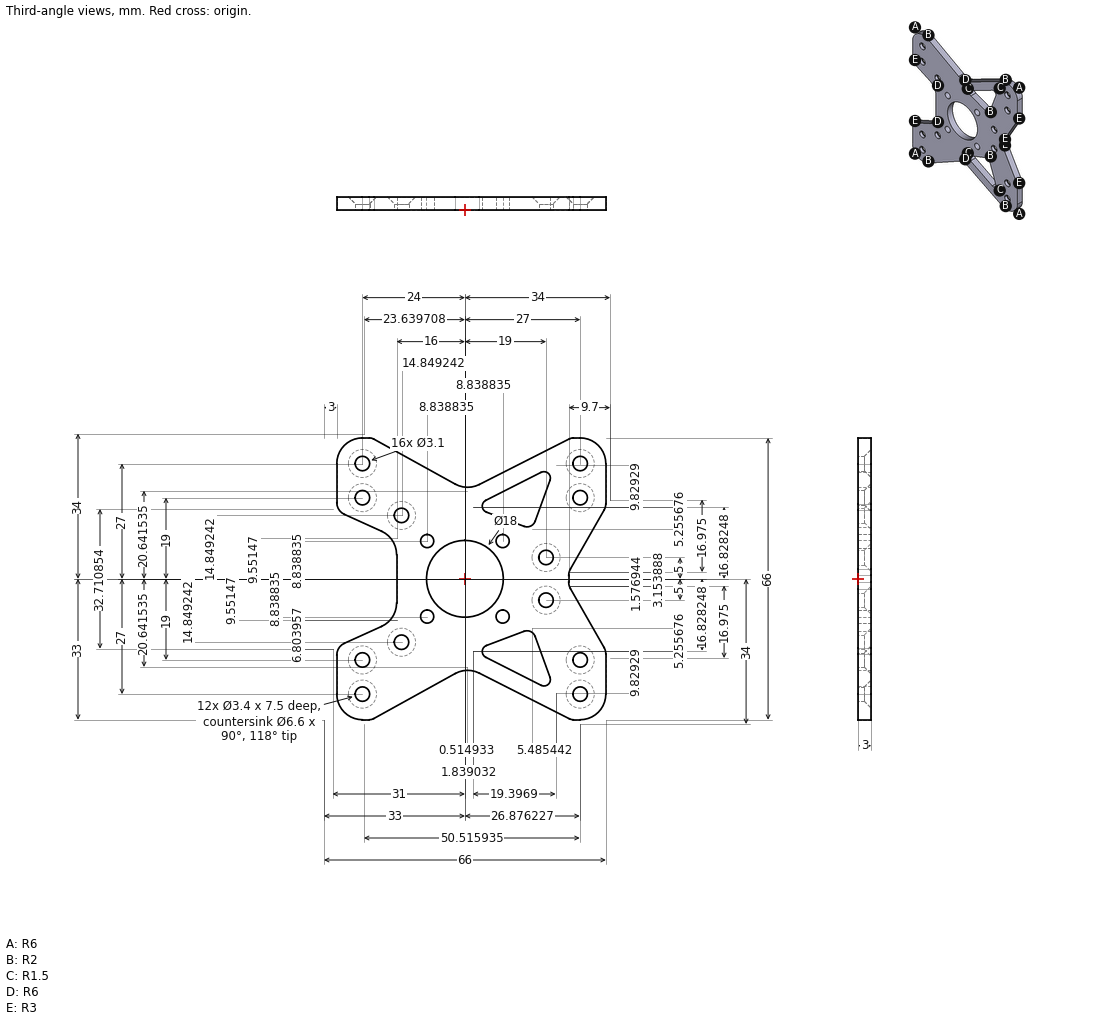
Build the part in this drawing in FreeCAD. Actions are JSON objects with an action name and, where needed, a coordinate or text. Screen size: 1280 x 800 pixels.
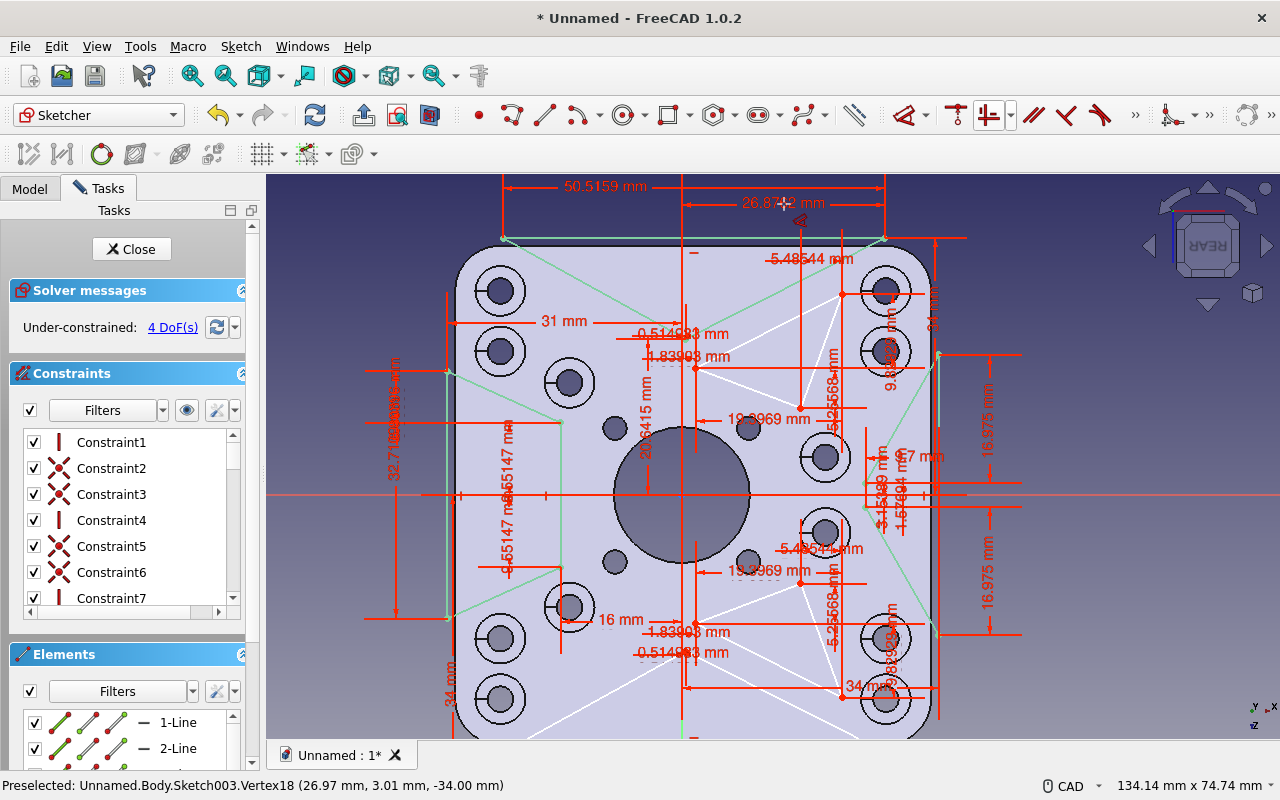
{"action": "left_click", "coordinate": [696, 368]}
{"action": "left_click", "coordinate": [648, 461]}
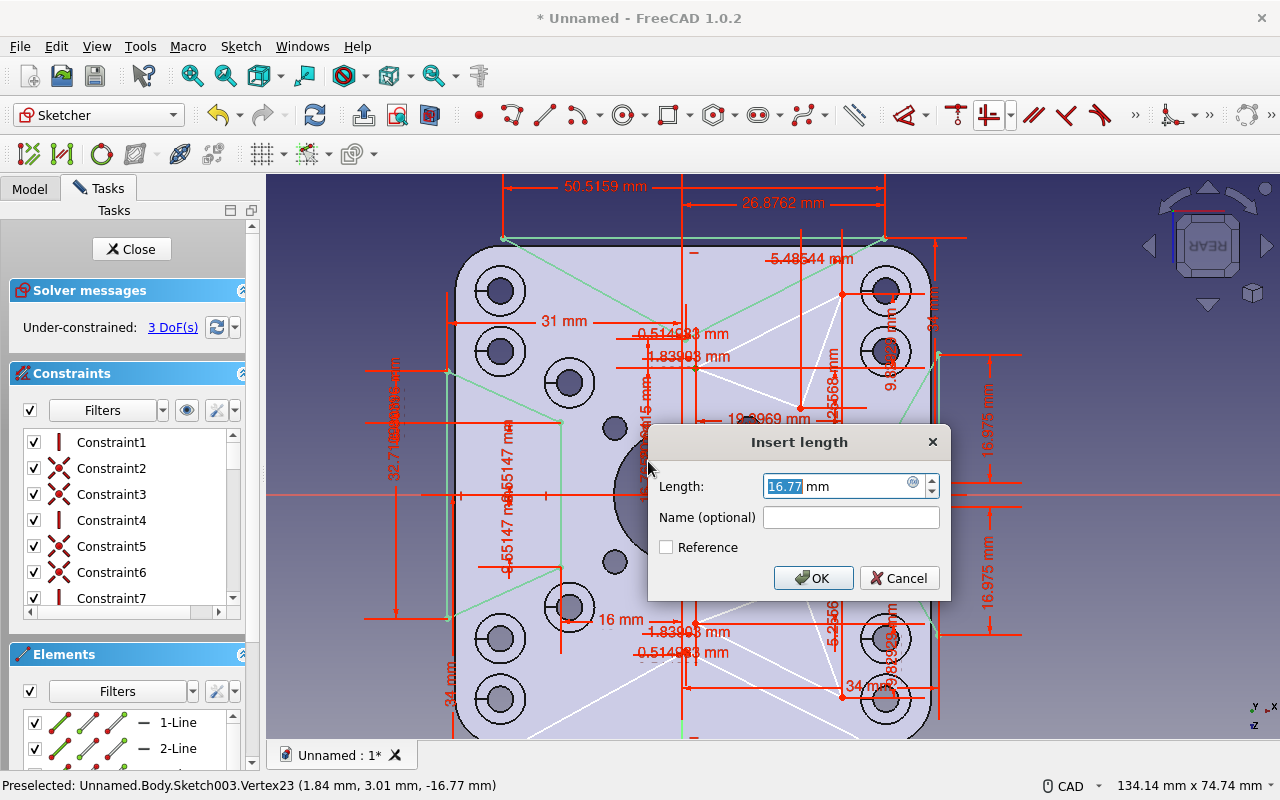
{"action": "type", "text": "16.828248"}
{"action": "key", "text": "Return"}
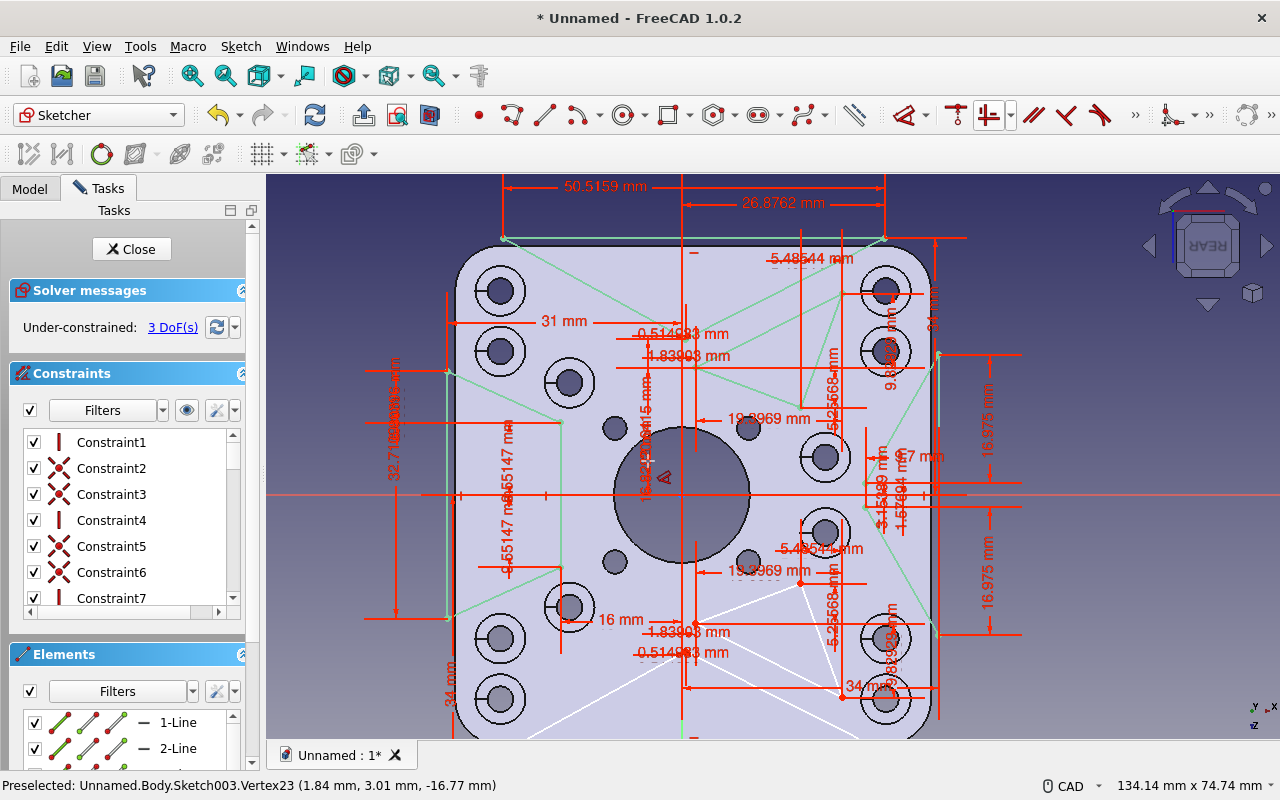
{"action": "left_click", "coordinate": [696, 624]}
{"action": "left_click", "coordinate": [648, 559]}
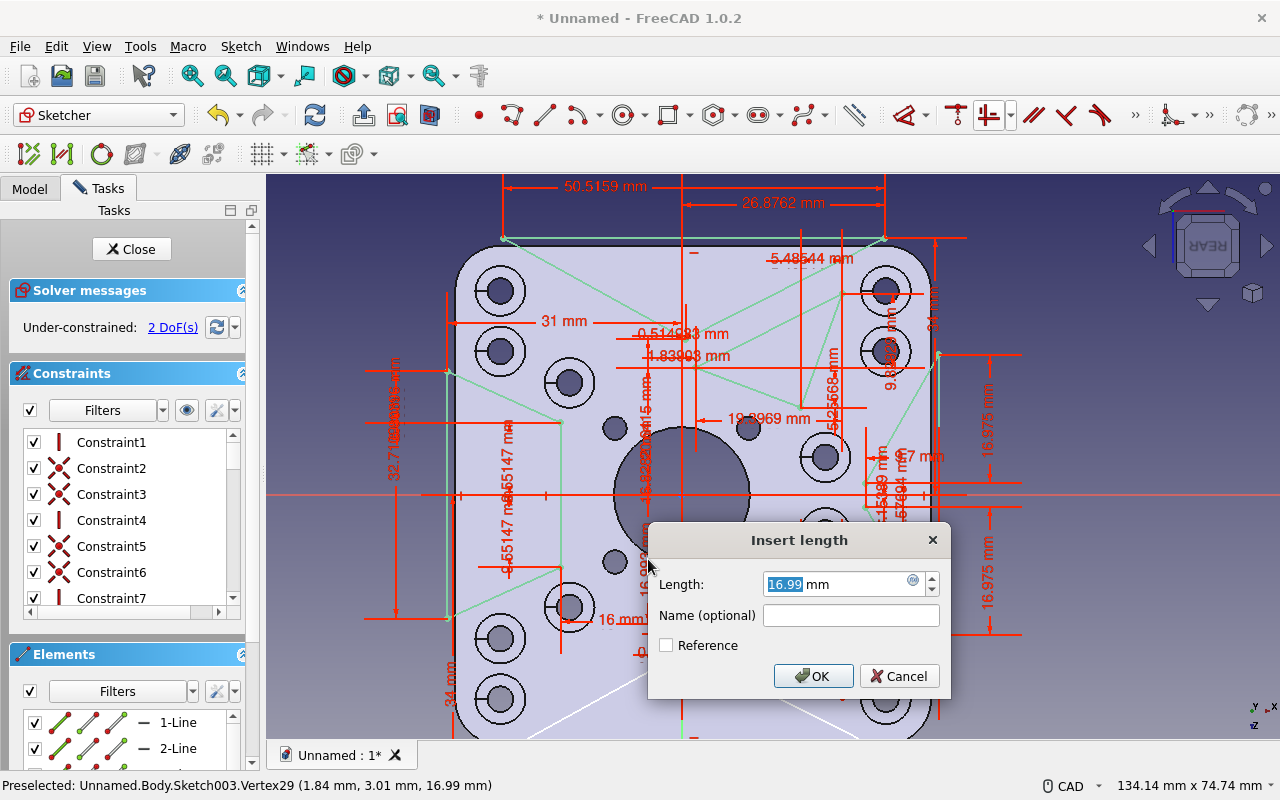
{"action": "type", "text": "16.828248"}
{"action": "key", "text": "Return"}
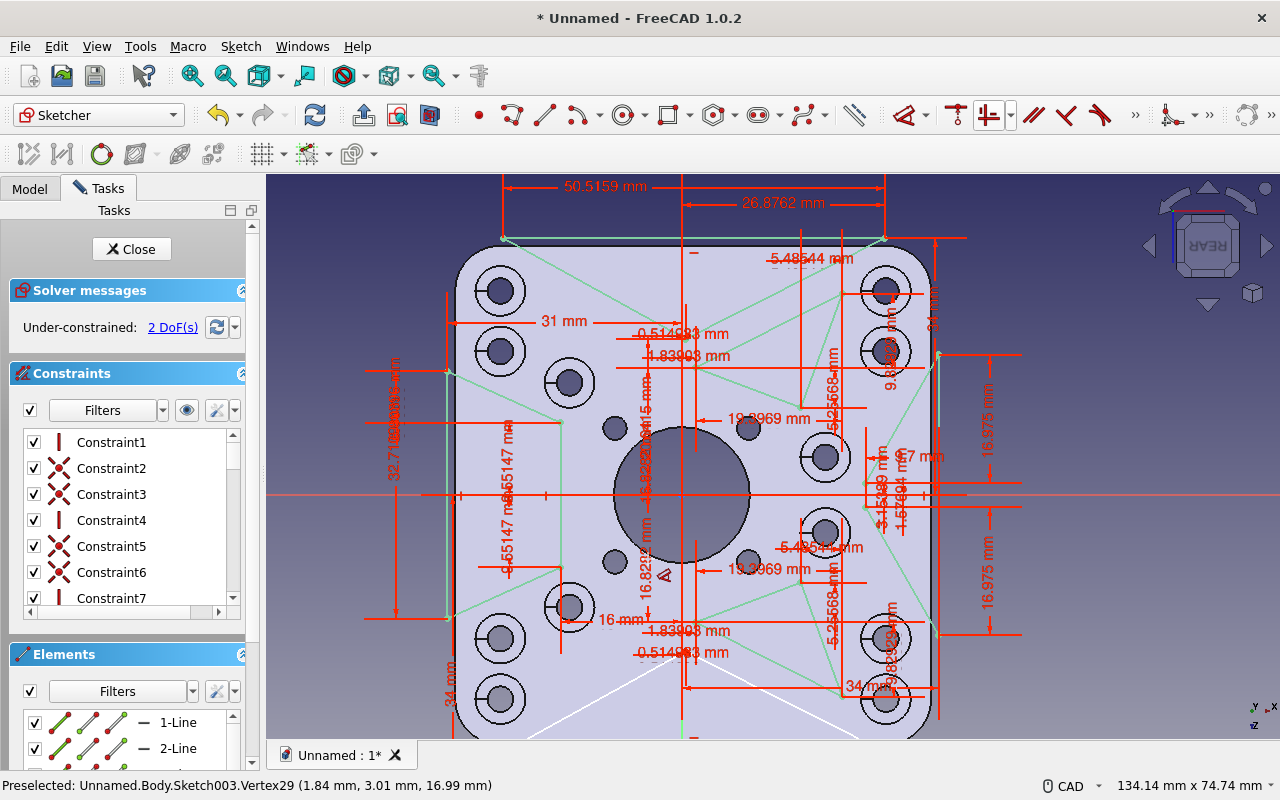
{"action": "left_click", "coordinate": [686, 651]}
{"action": "left_click", "coordinate": [648, 537]}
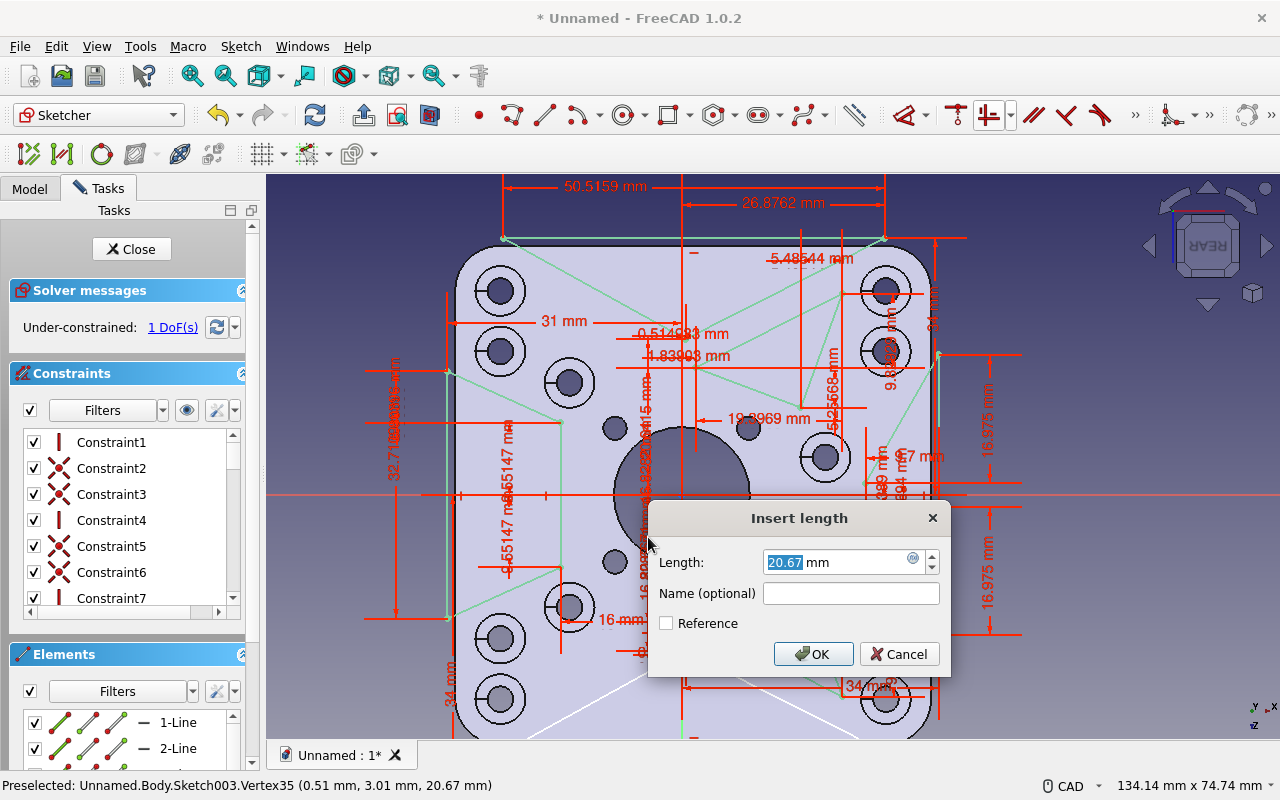
{"action": "type", "text": "20.641535"}
{"action": "key", "text": "Return"}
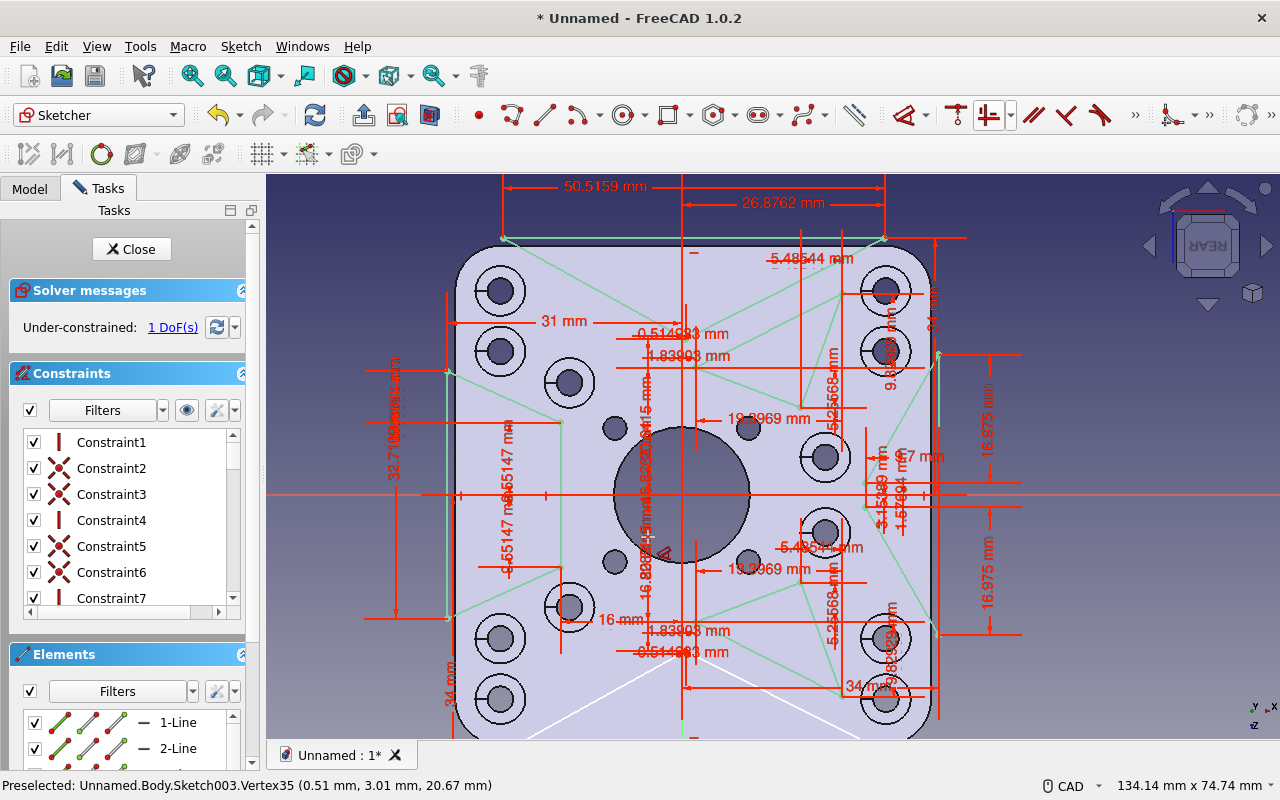
{"action": "scroll", "coordinate": [728, 378], "scroll_direction": "down", "scroll_amount": 2}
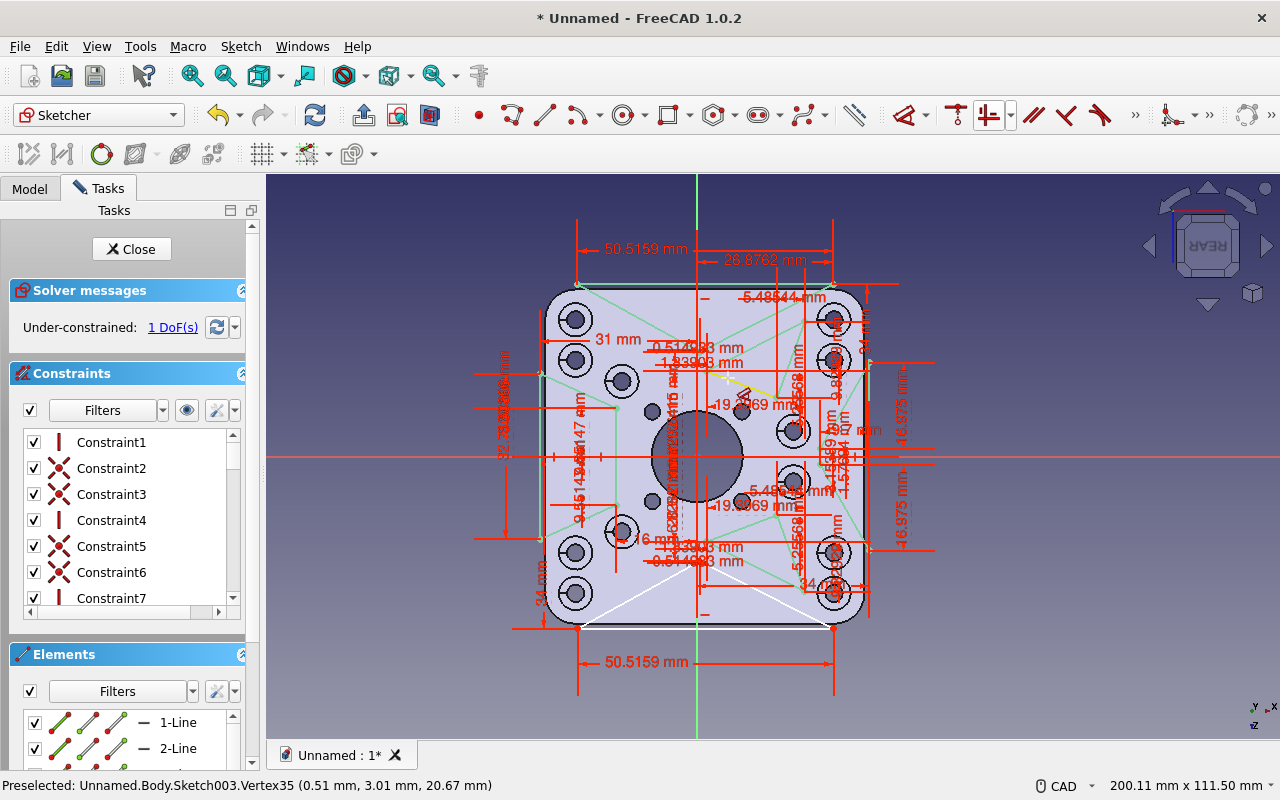
{"action": "left_click", "coordinate": [578, 629]}
{"action": "left_click", "coordinate": [637, 687]}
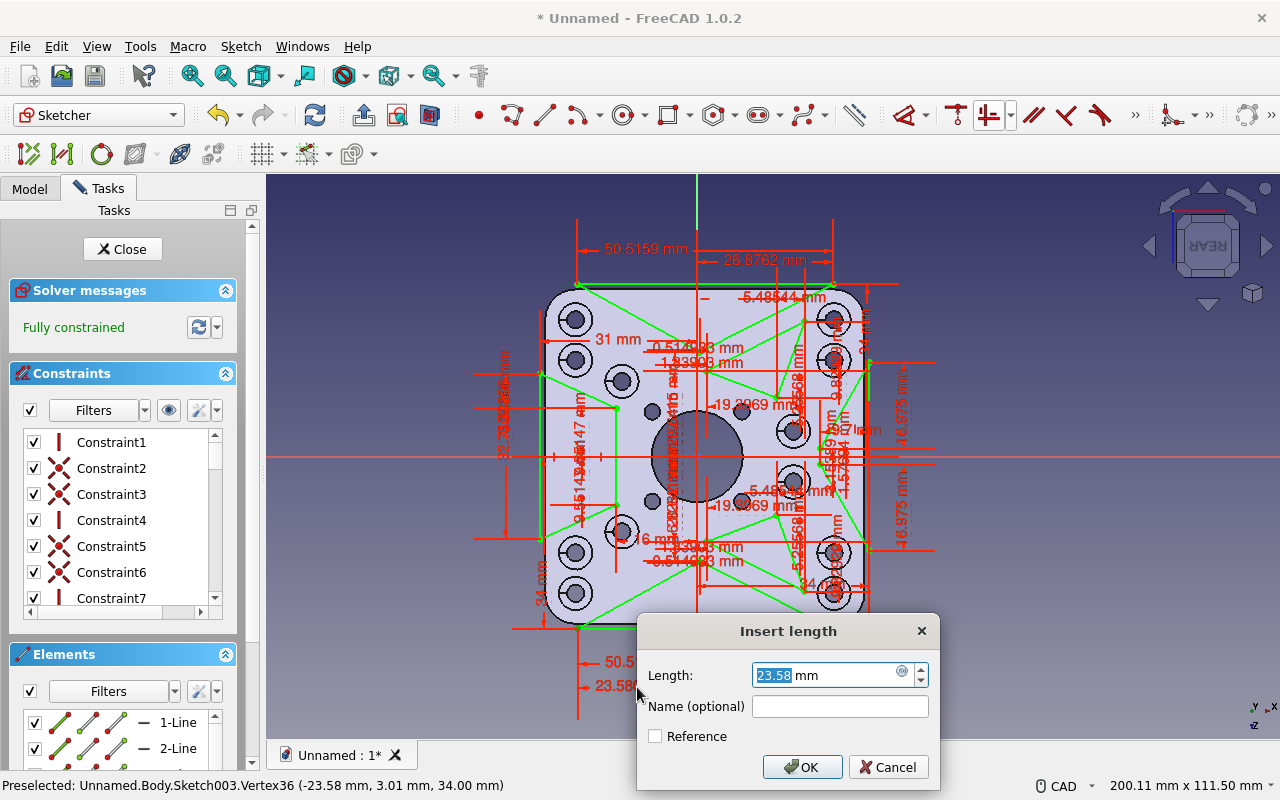
{"action": "type", "text": "23.639708"}
{"action": "key", "text": "Return"}
{"action": "key", "text": "Escape"}